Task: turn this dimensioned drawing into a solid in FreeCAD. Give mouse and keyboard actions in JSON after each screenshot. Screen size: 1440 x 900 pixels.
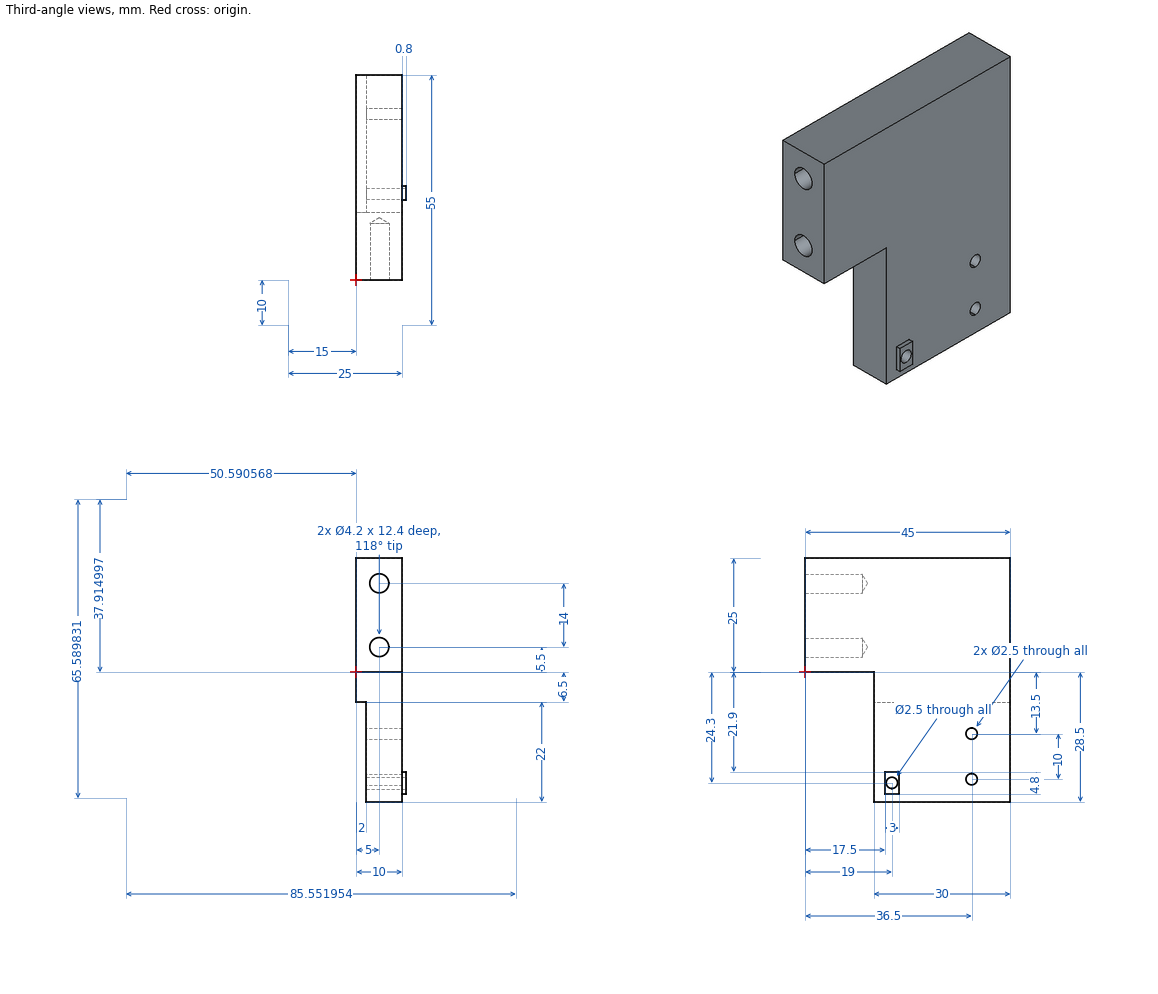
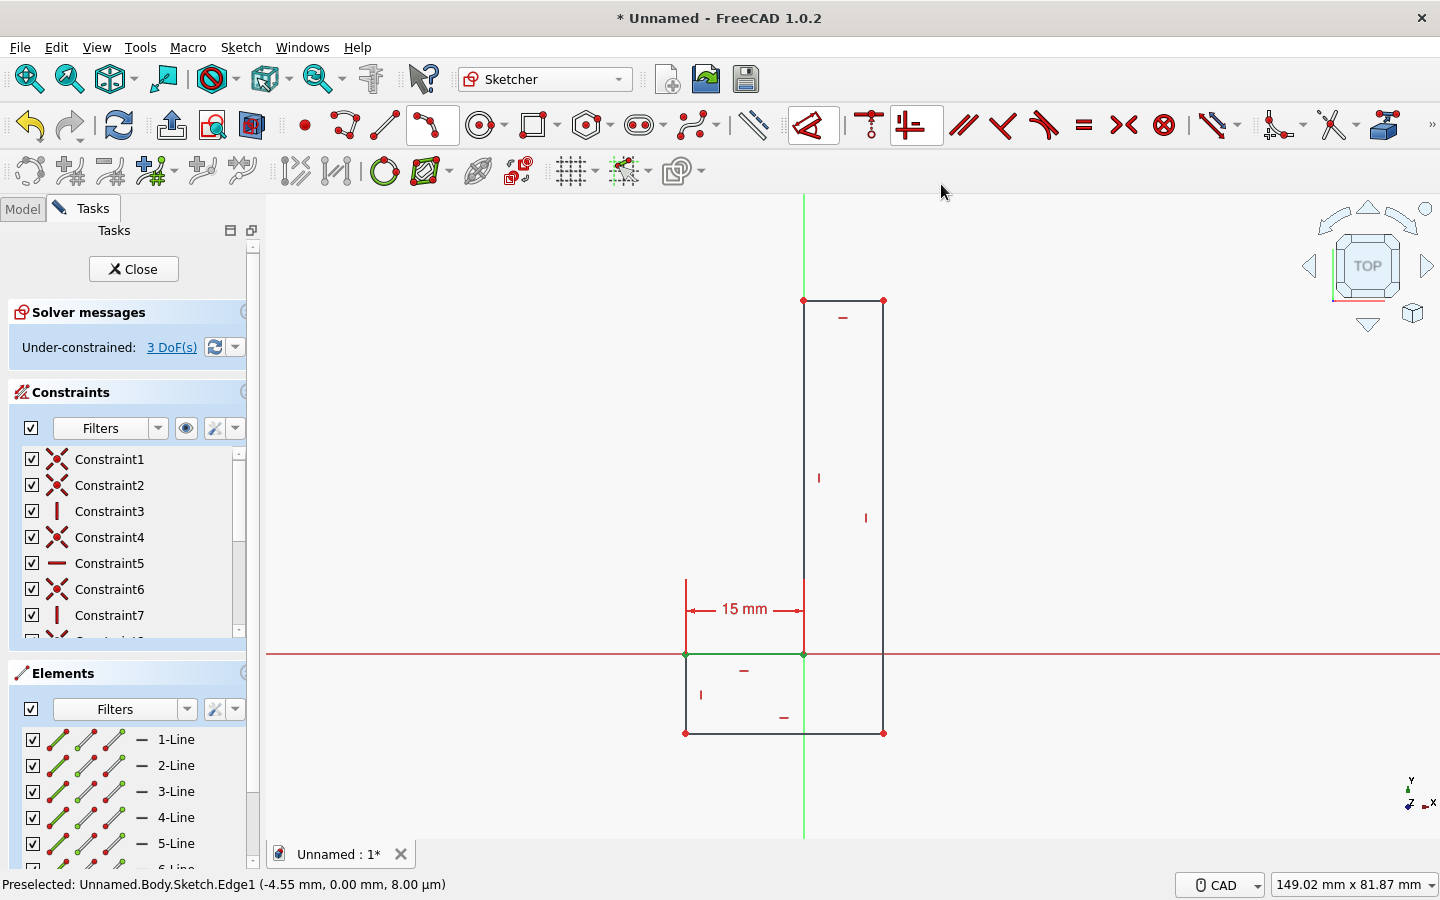
{"action": "left_click", "coordinate": [686, 678]}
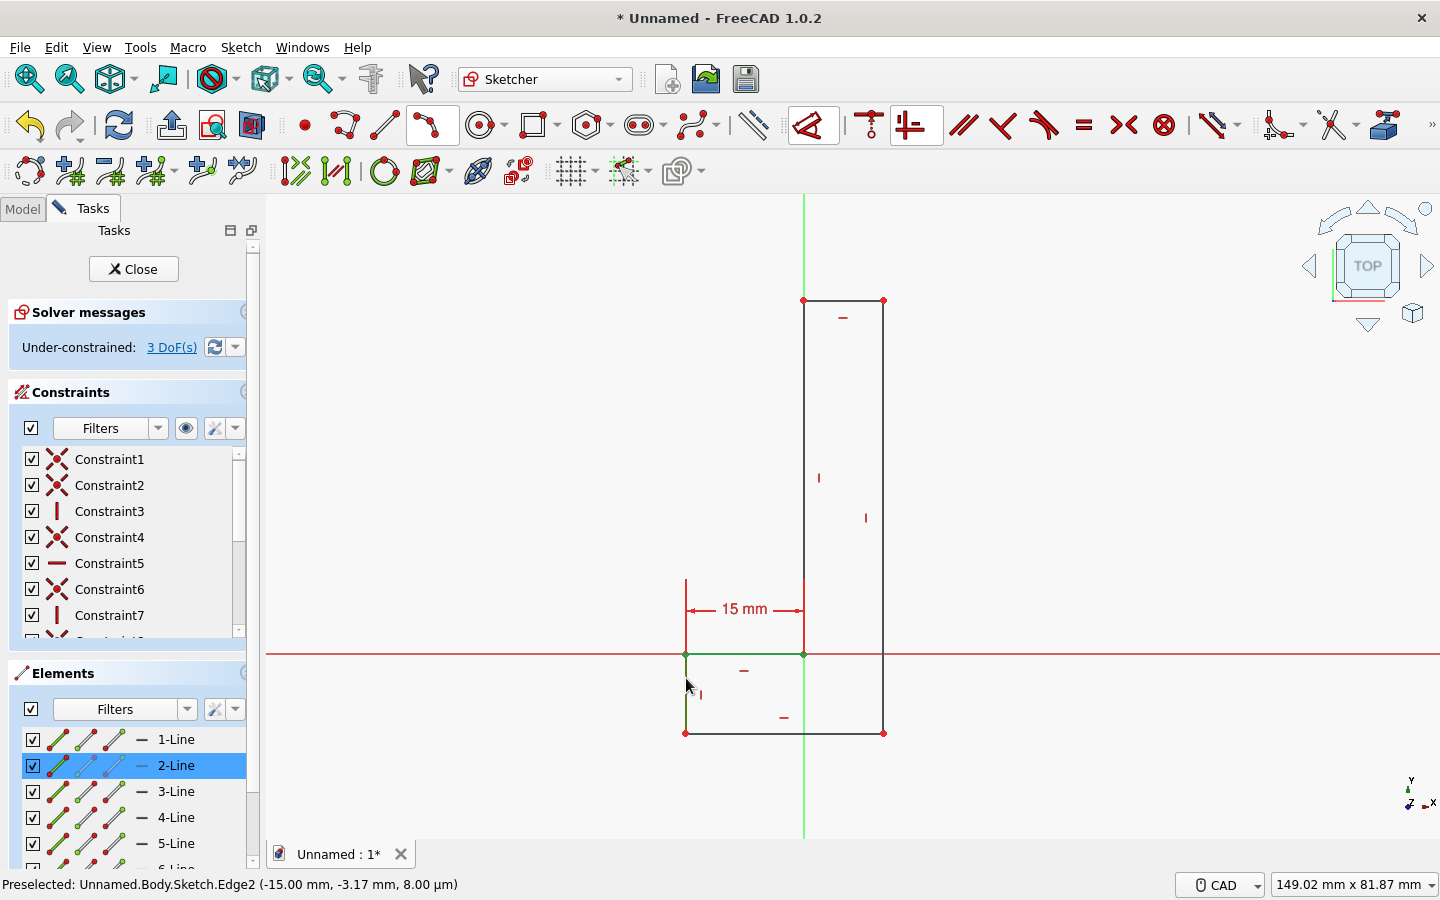
{"action": "left_click", "coordinate": [834, 126]}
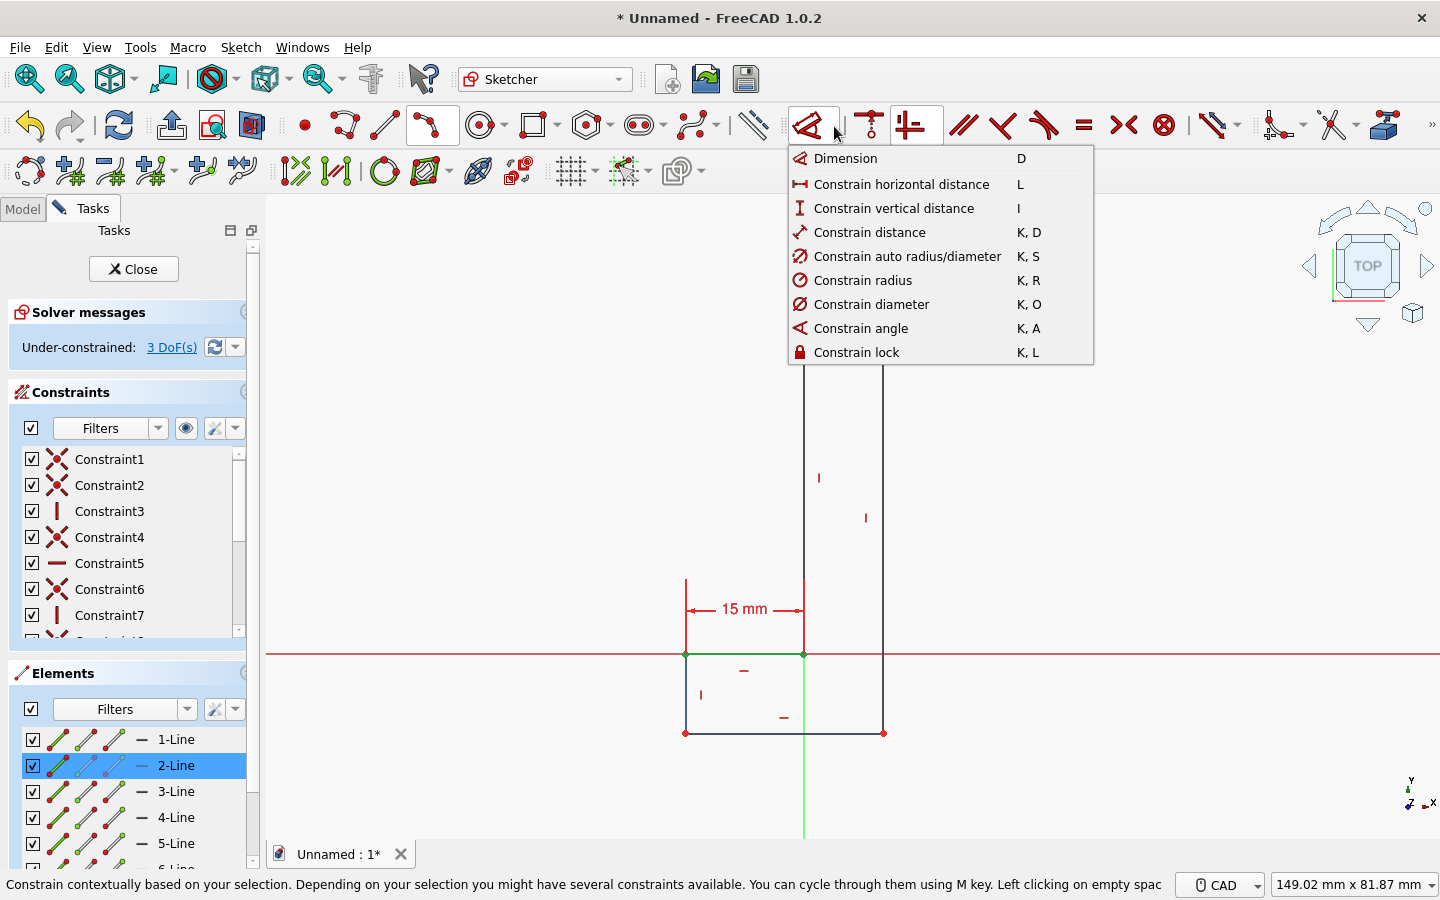
{"action": "left_click", "coordinate": [941, 208]}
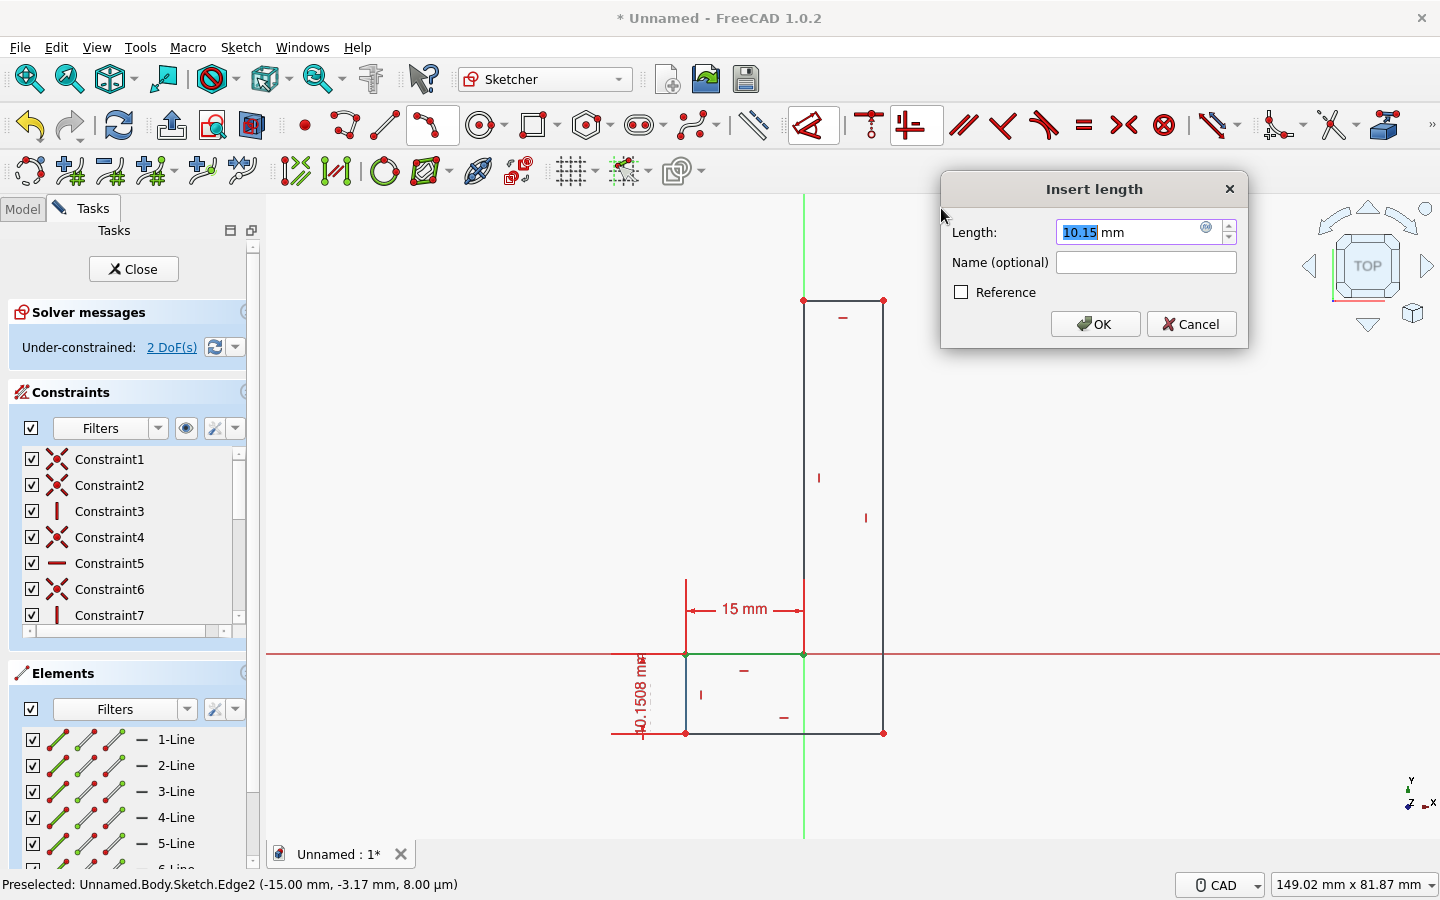
{"action": "type", "text": "10"}
{"action": "key", "text": "Return"}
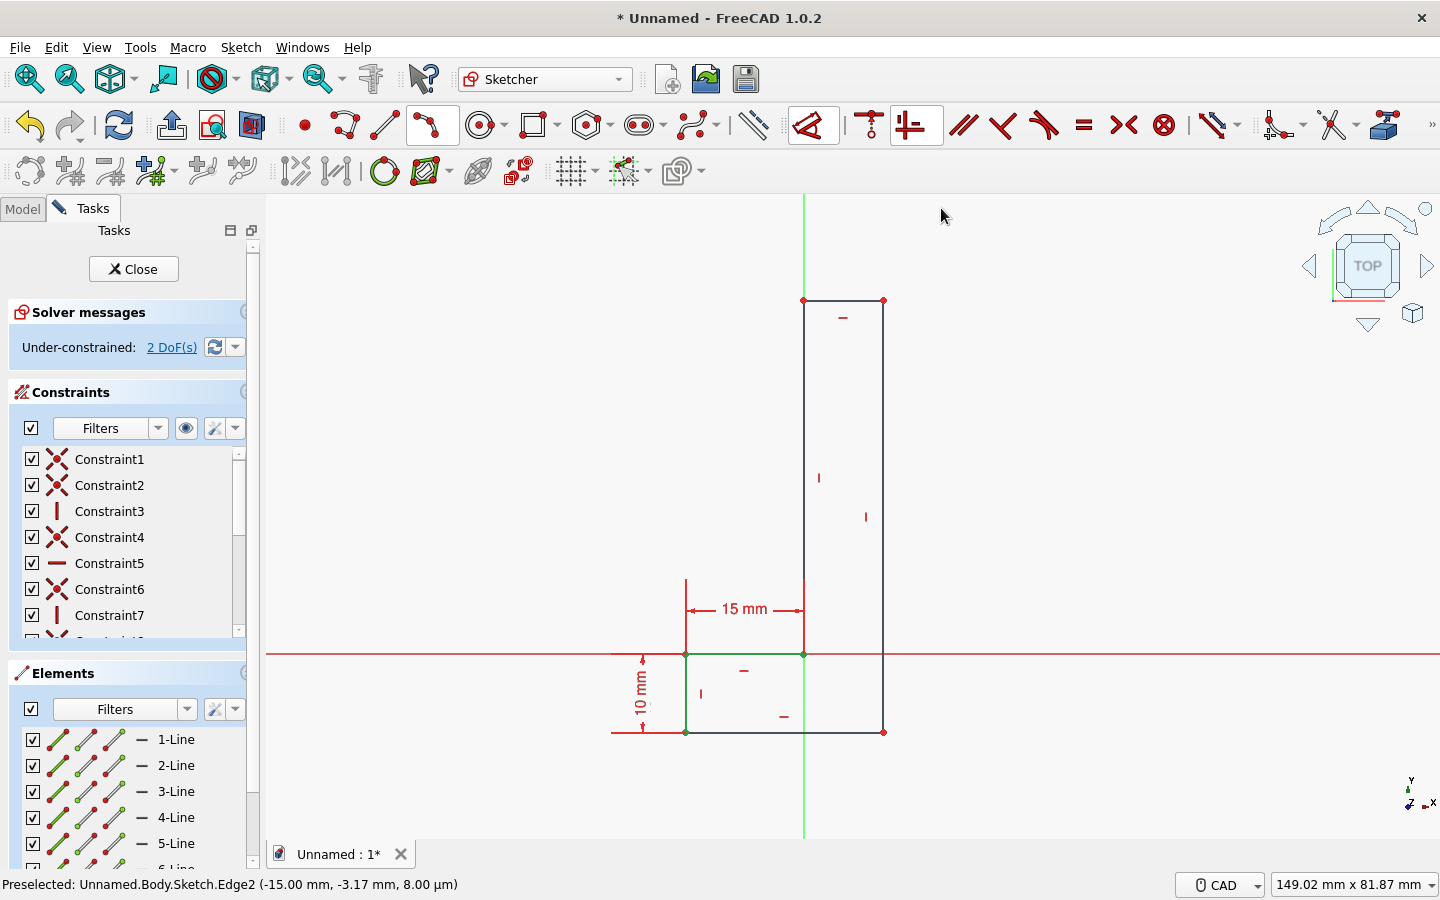
{"action": "left_click", "coordinate": [745, 733]}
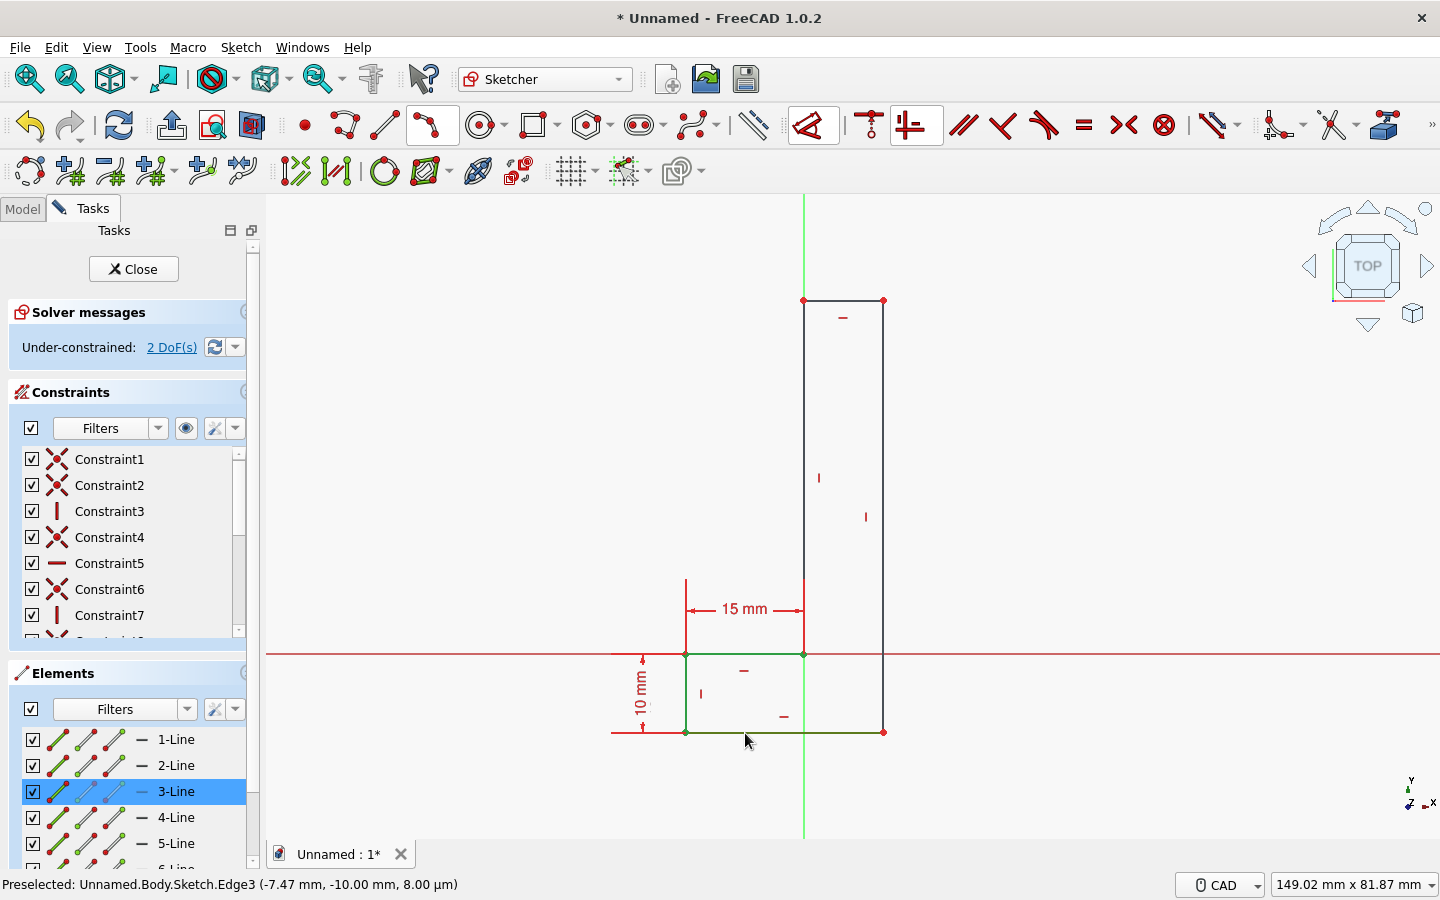
{"action": "left_click", "coordinate": [834, 126]}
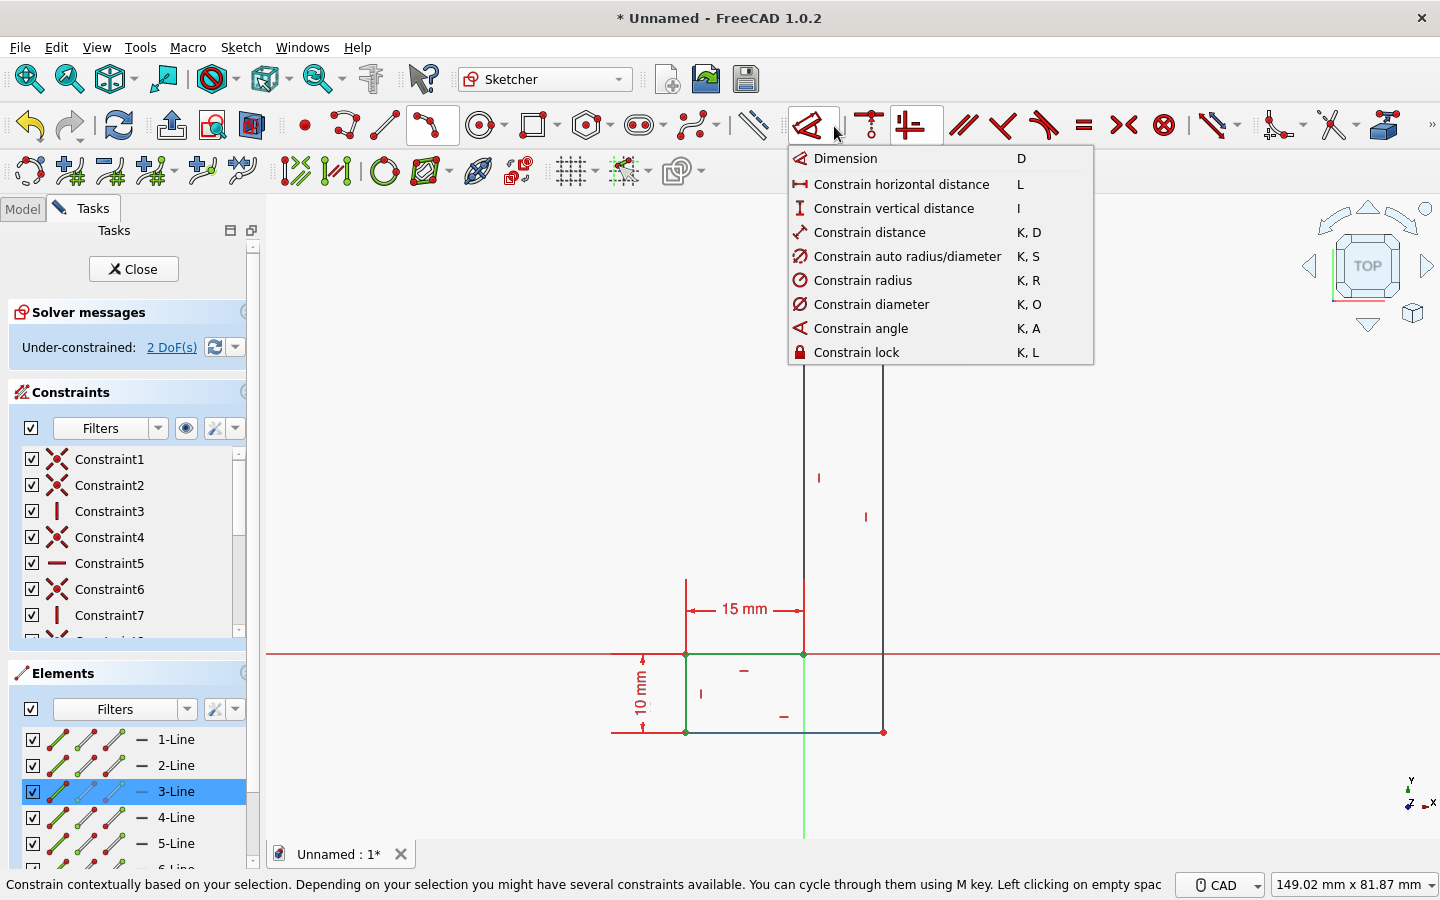
{"action": "left_click", "coordinate": [941, 184]}